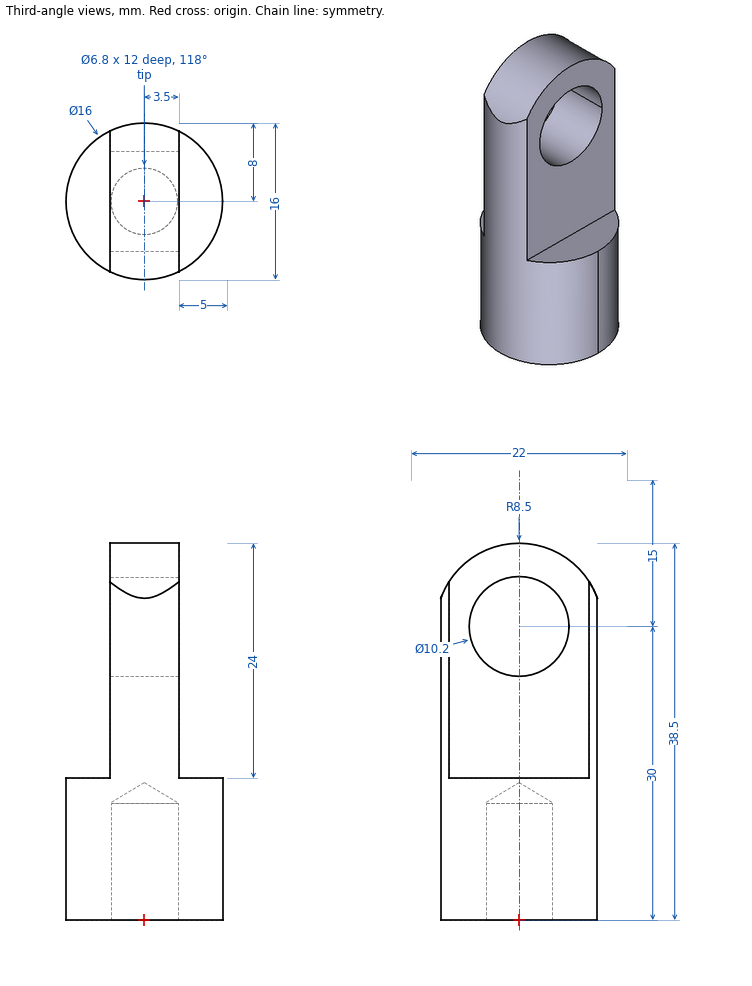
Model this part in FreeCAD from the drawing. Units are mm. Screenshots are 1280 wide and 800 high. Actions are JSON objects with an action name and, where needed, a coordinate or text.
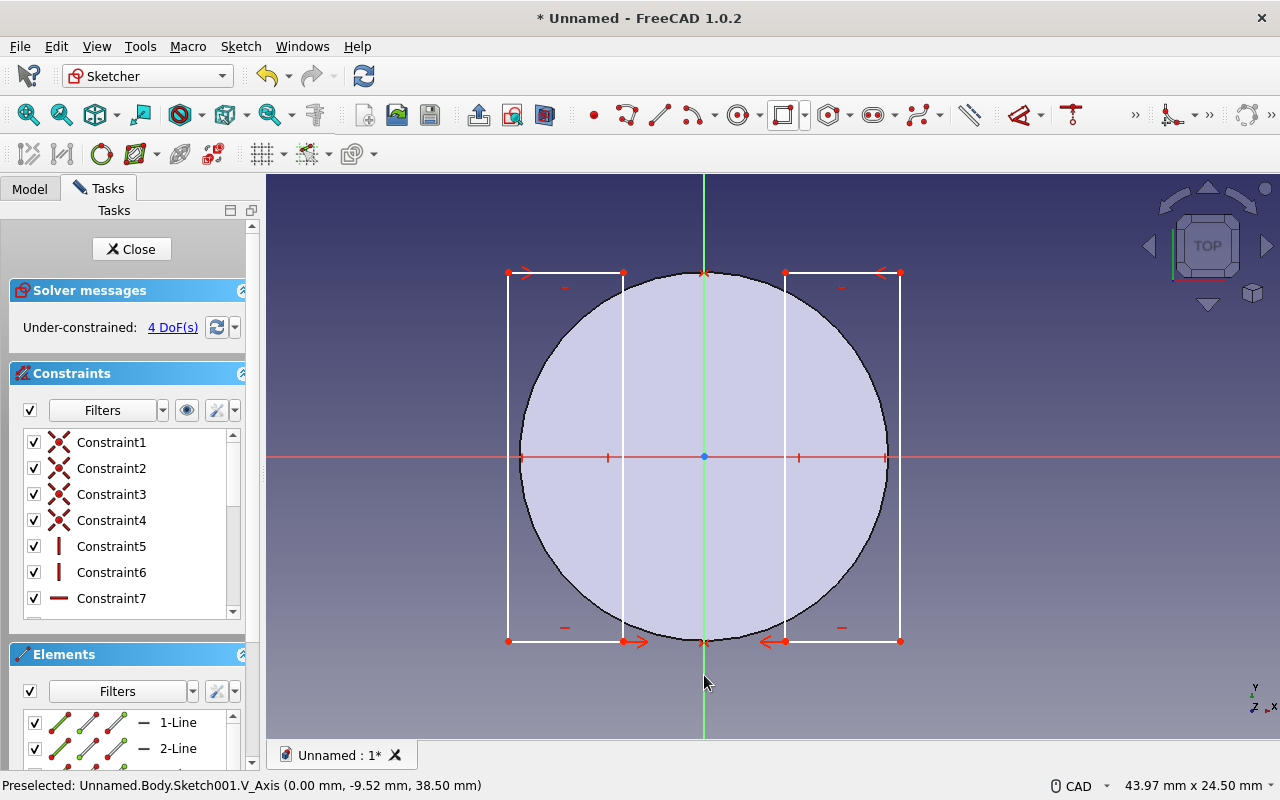
{"action": "key", "text": "d"}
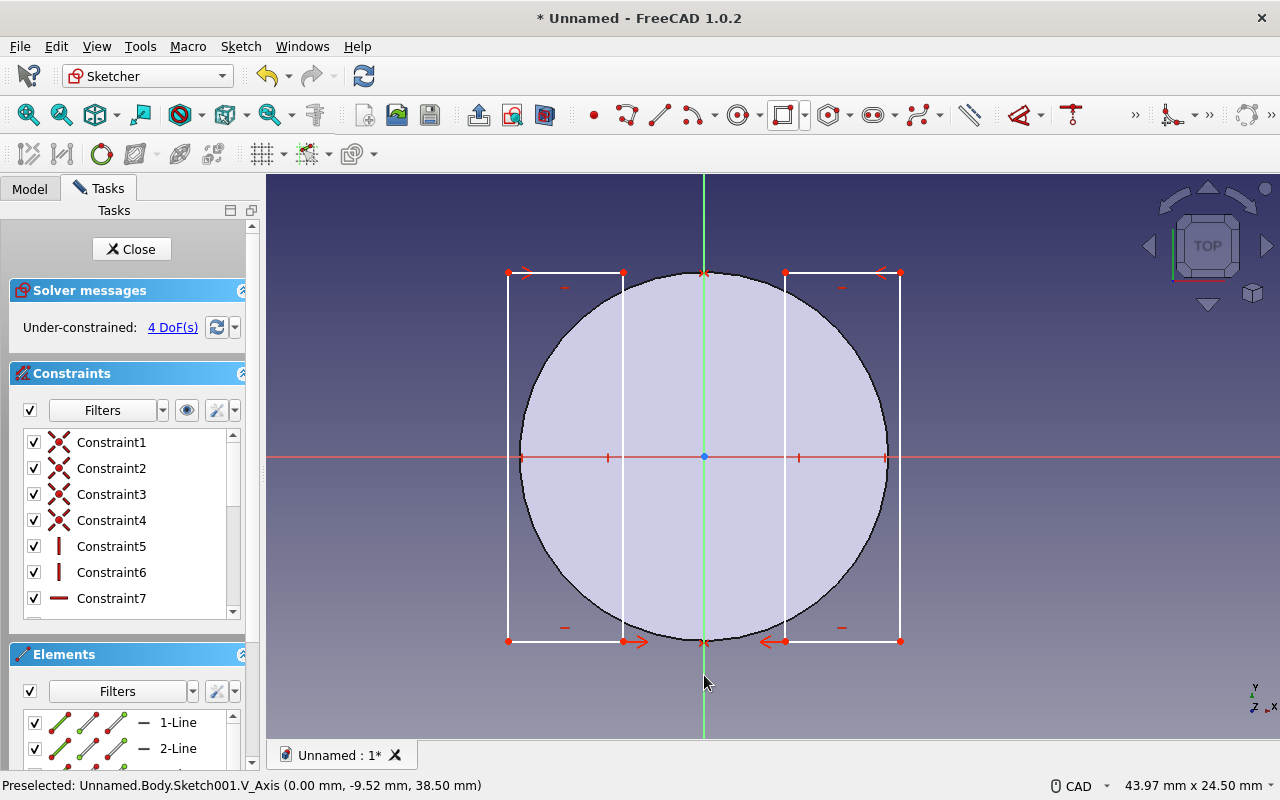
{"action": "left_click", "coordinate": [820, 642]}
{"action": "left_click", "coordinate": [843, 676]}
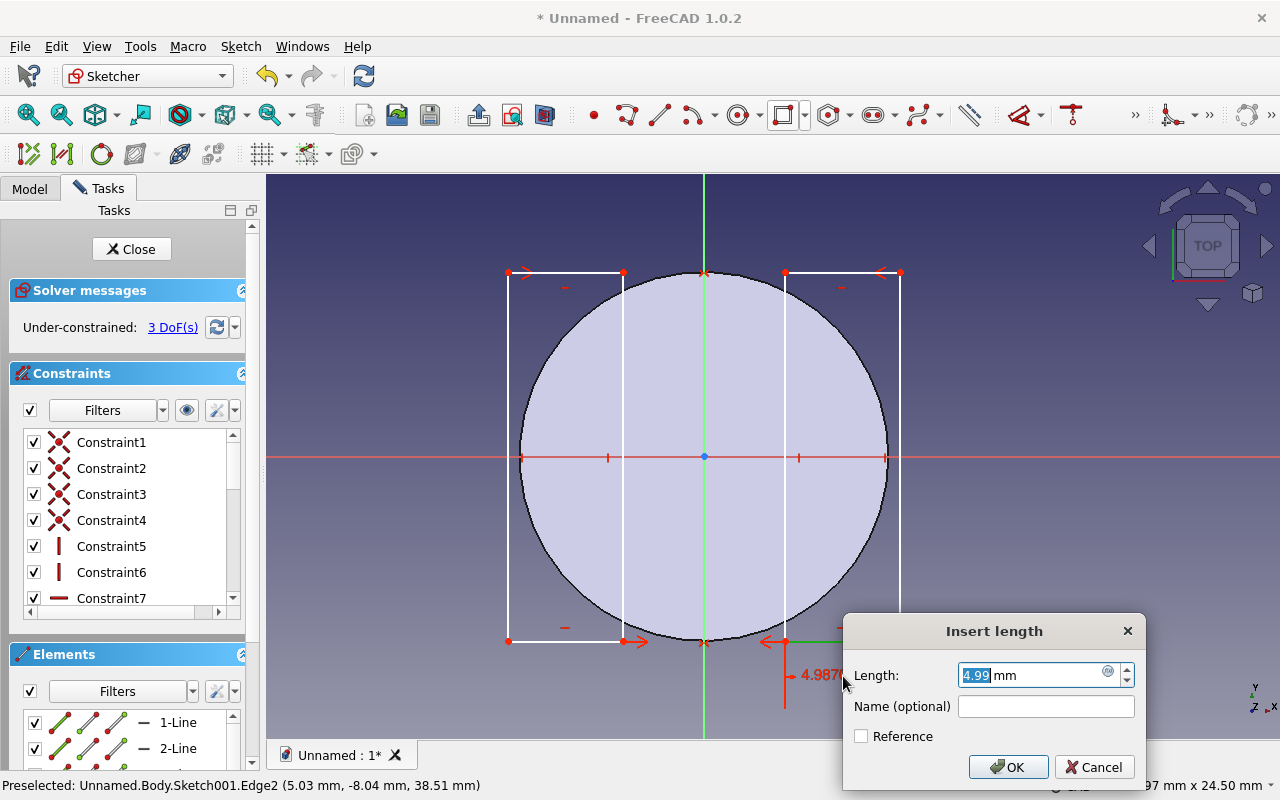
{"action": "type", "text": "5"}
{"action": "key", "text": "Return"}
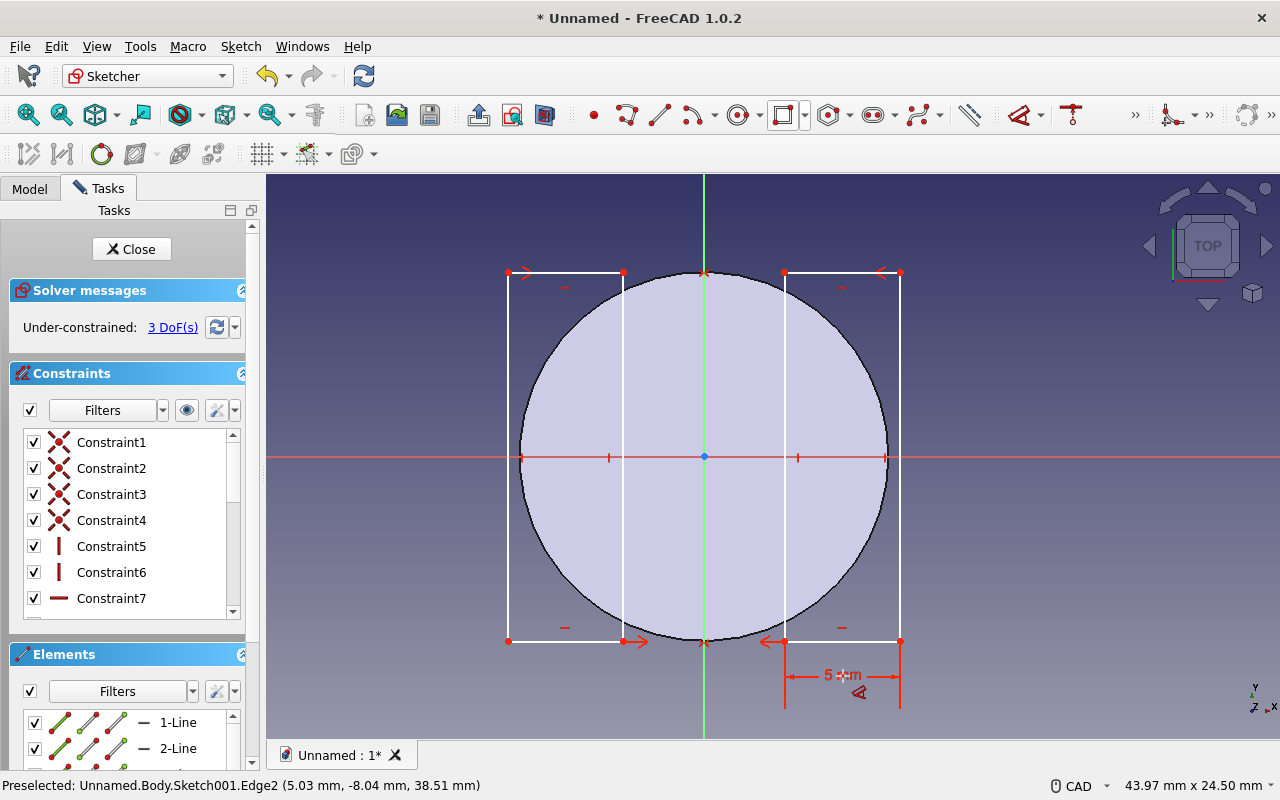
{"action": "left_click", "coordinate": [785, 384]}
{"action": "left_click", "coordinate": [819, 373]}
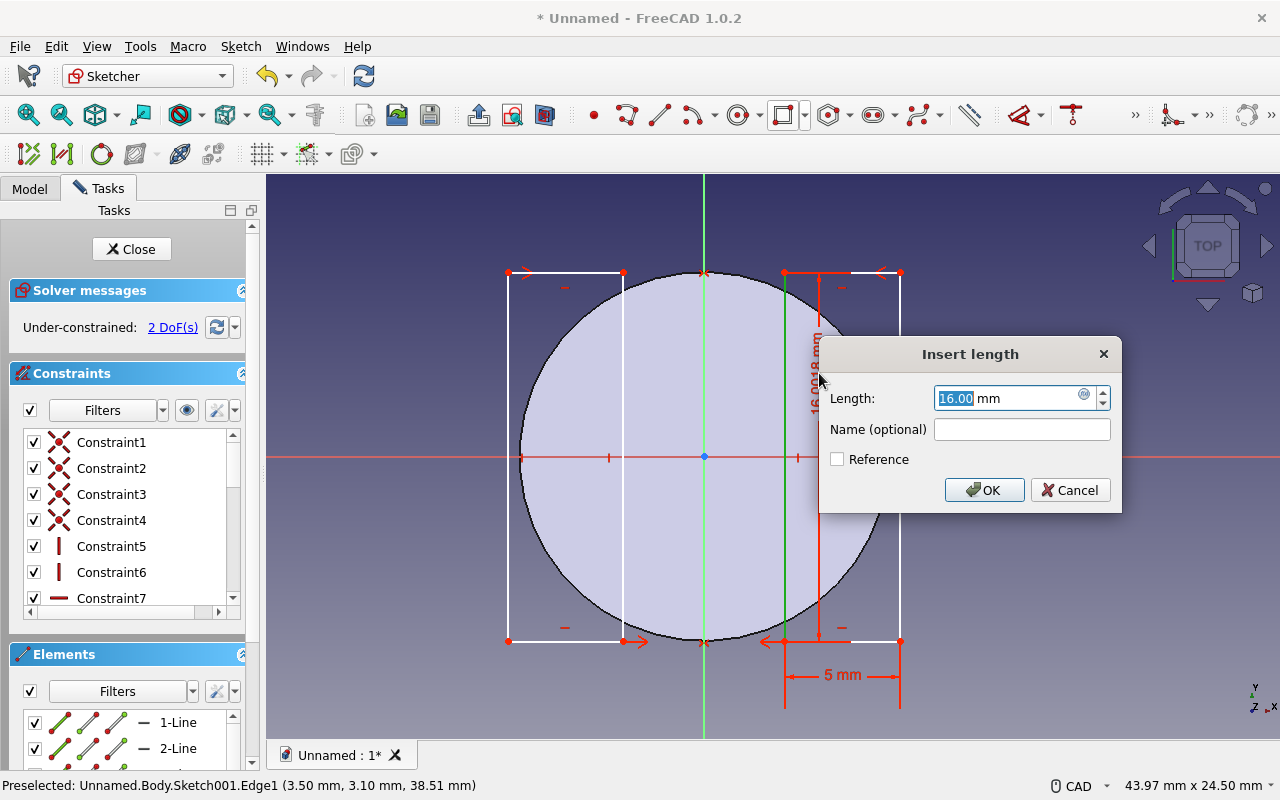
{"action": "type", "text": "16"}
{"action": "key", "text": "Return"}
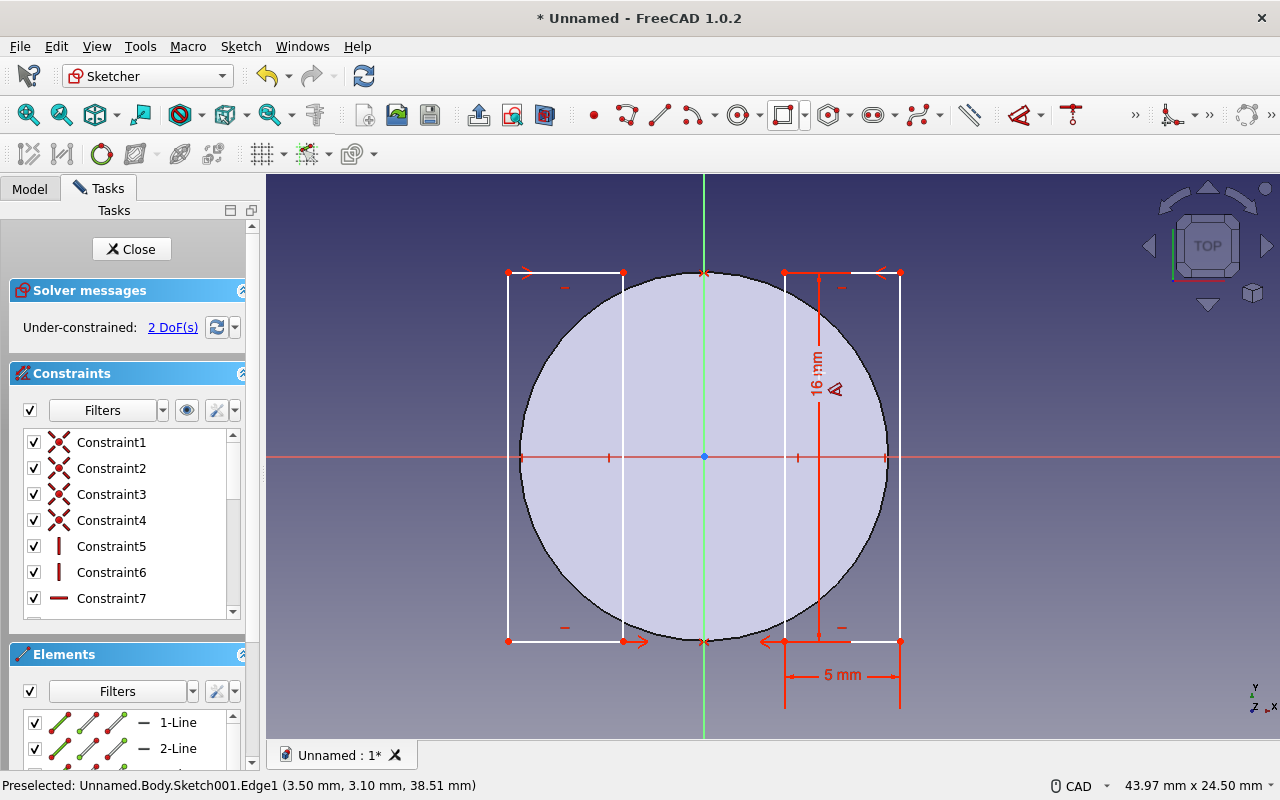
{"action": "left_click", "coordinate": [785, 273]}
{"action": "left_click", "coordinate": [819, 323]}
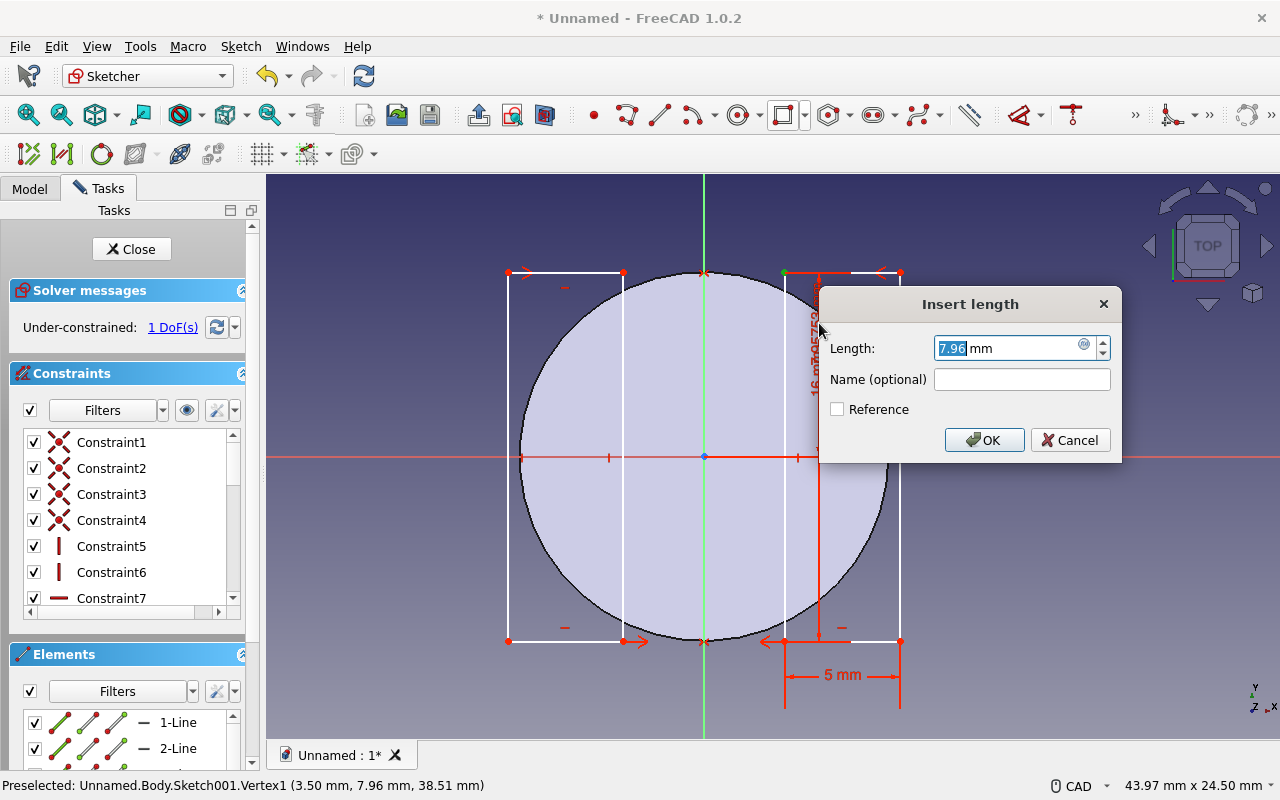
{"action": "type", "text": "8"}
{"action": "key", "text": "Return"}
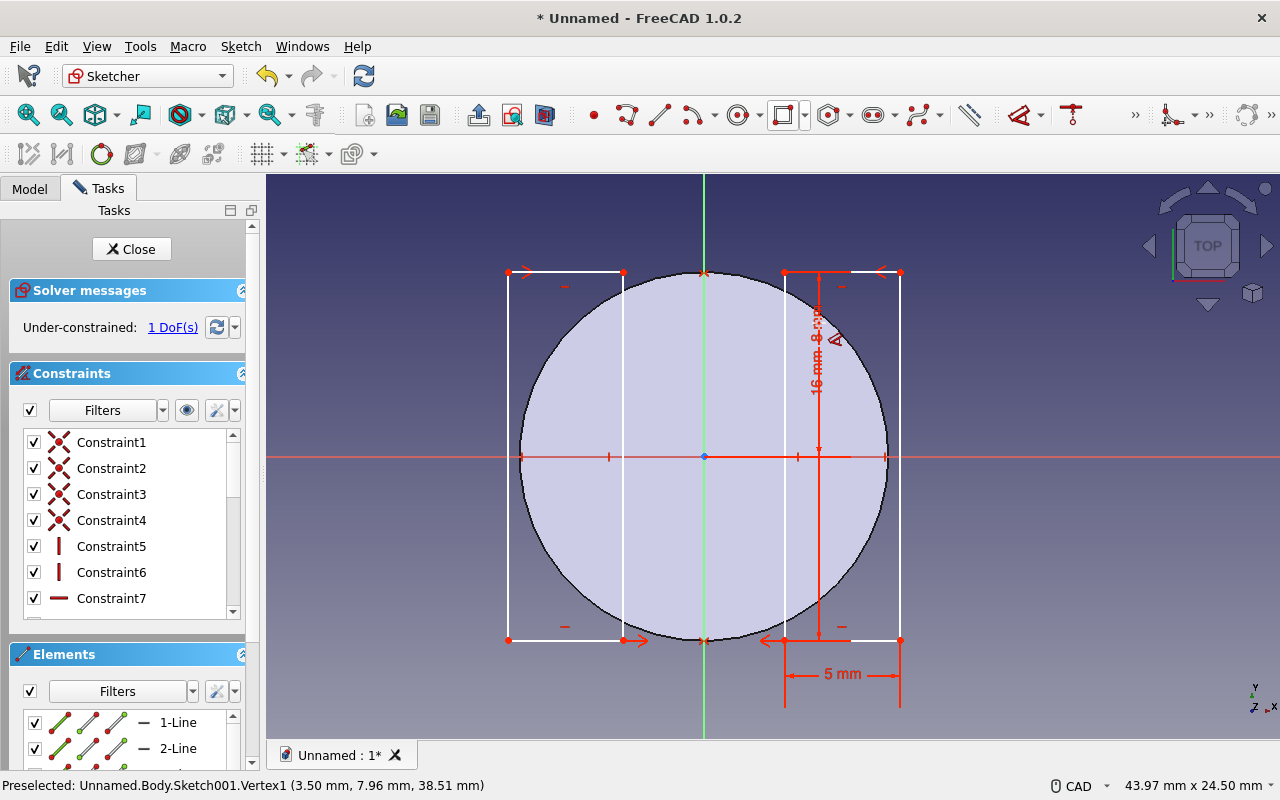
{"action": "left_click", "coordinate": [785, 272]}
{"action": "left_click", "coordinate": [744, 238]}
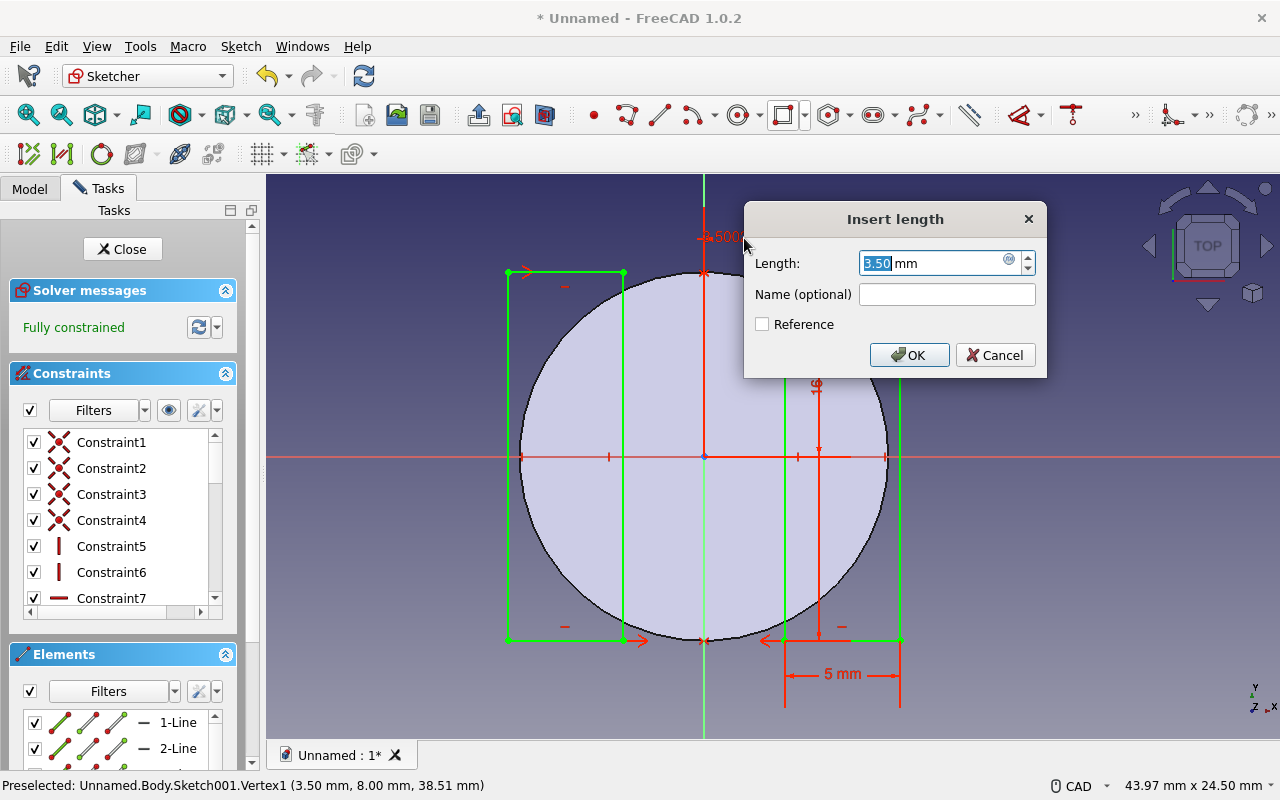
{"action": "type", "text": "3.5"}
{"action": "key", "text": "Return"}
{"action": "key", "text": "Escape"}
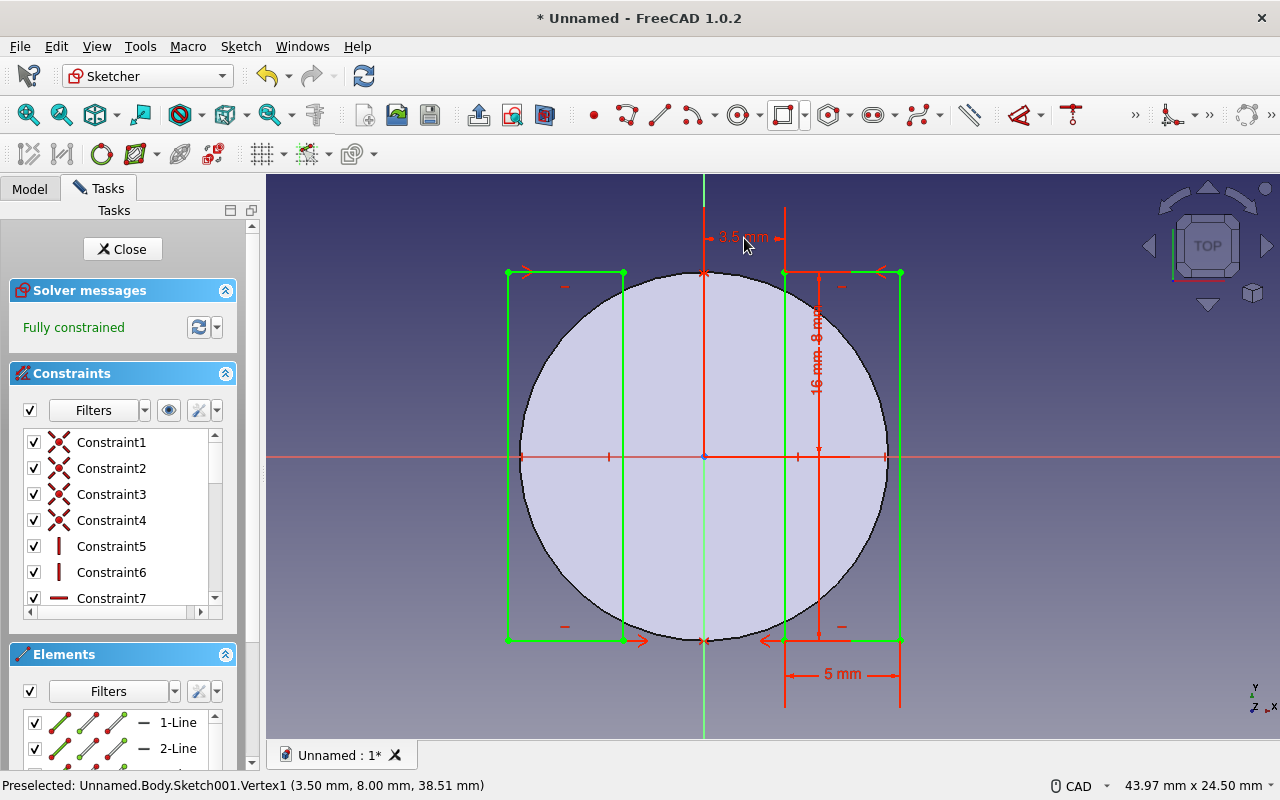
{"action": "left_click", "coordinate": [123, 249]}